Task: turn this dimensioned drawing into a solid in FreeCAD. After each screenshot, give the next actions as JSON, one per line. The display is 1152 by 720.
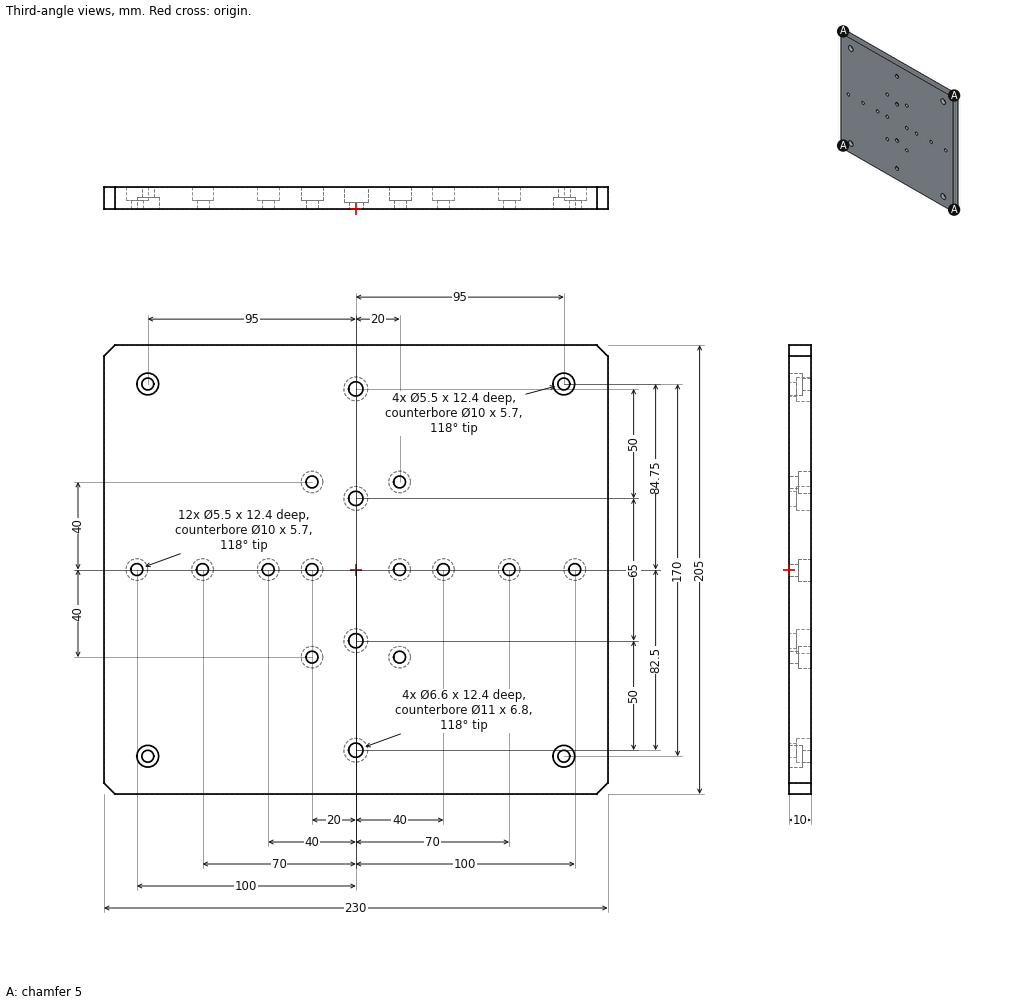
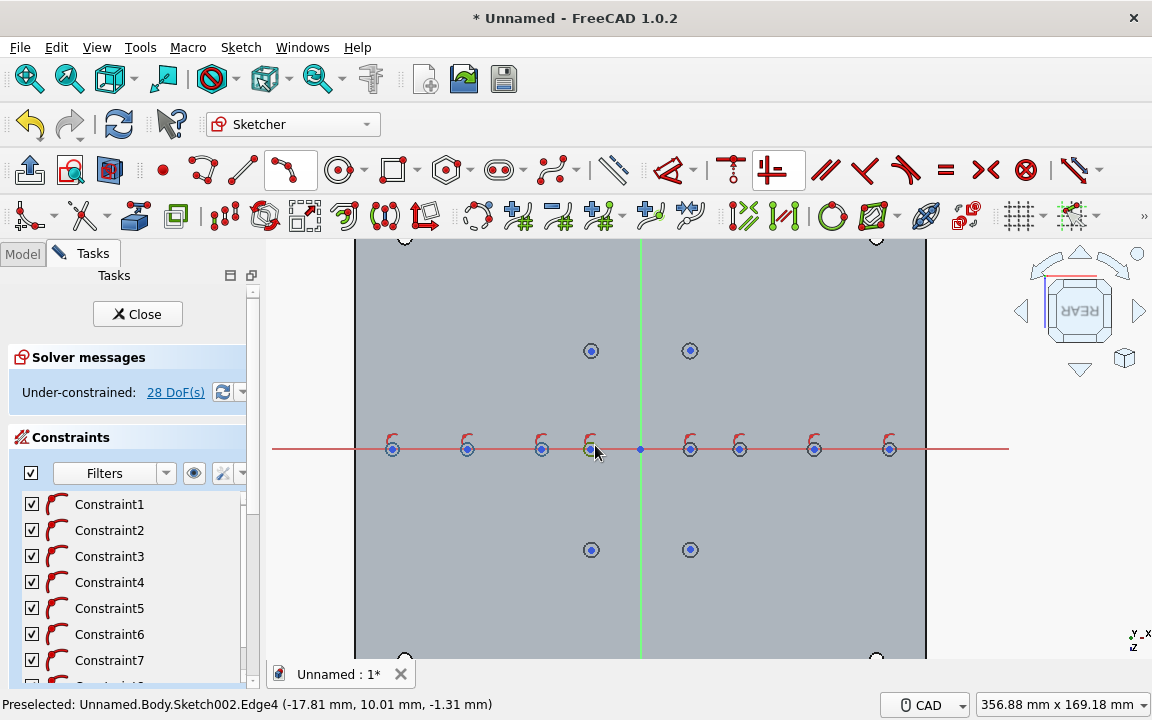
{"action": "scroll", "coordinate": [596, 346], "scroll_direction": "up", "scroll_amount": 4}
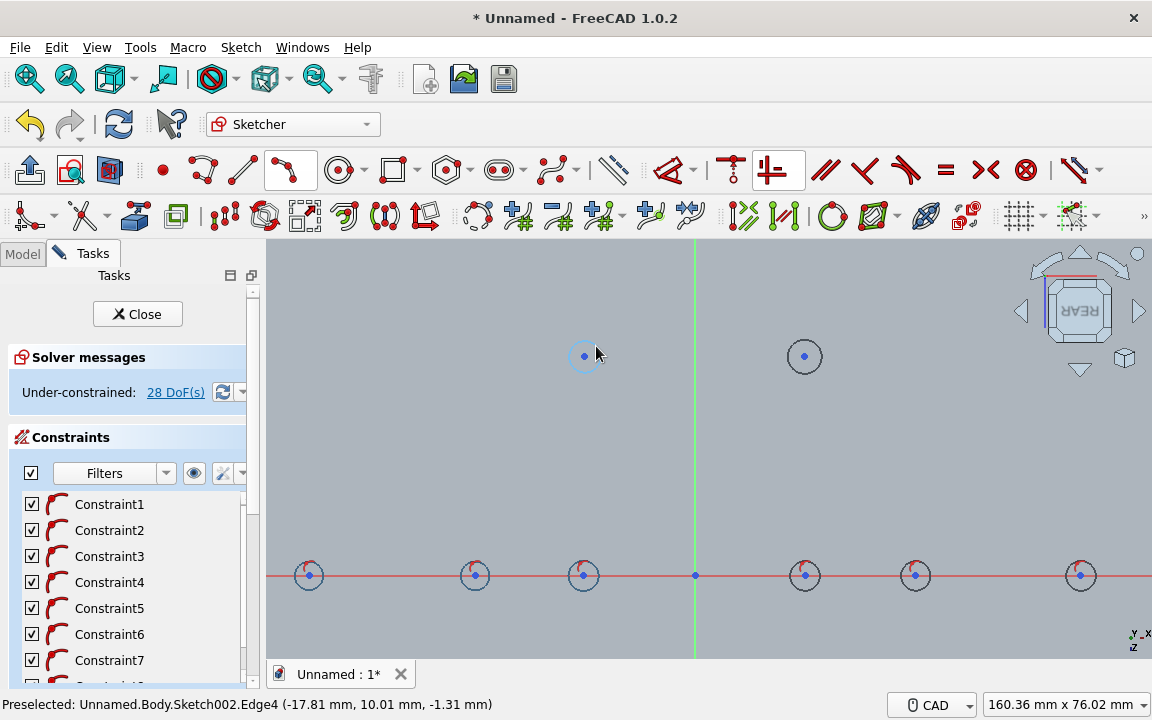
{"action": "left_click", "coordinate": [596, 346]}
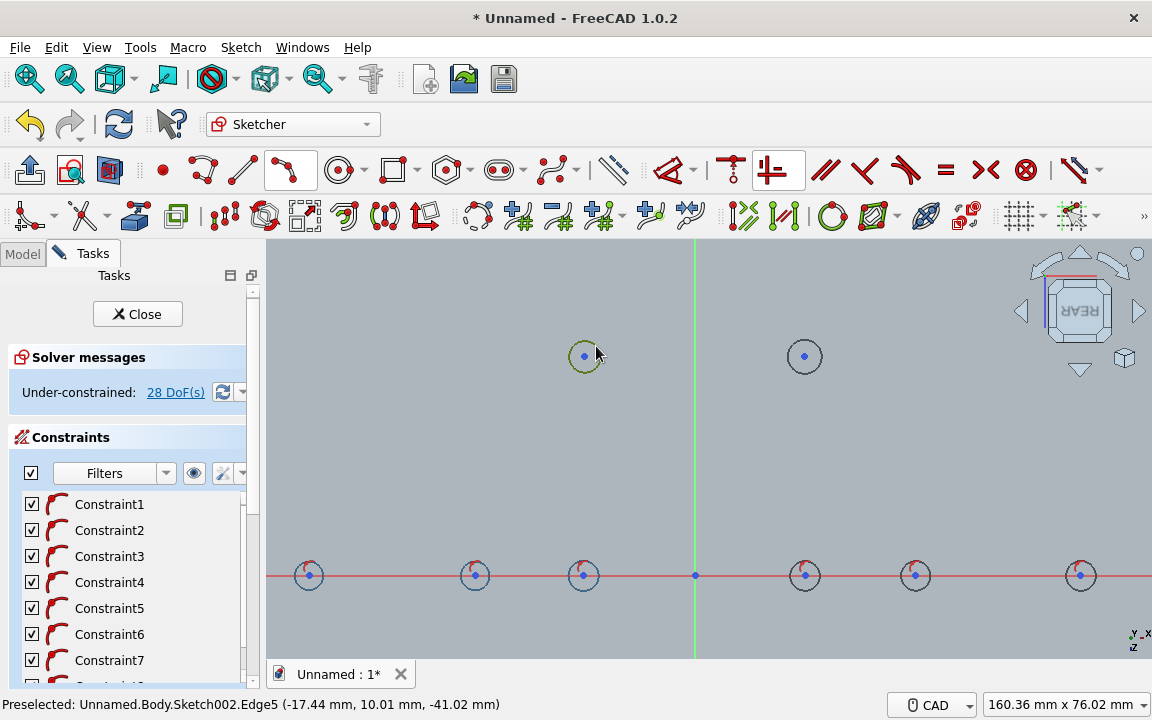
{"action": "scroll", "coordinate": [596, 345], "scroll_direction": "down", "scroll_amount": 4}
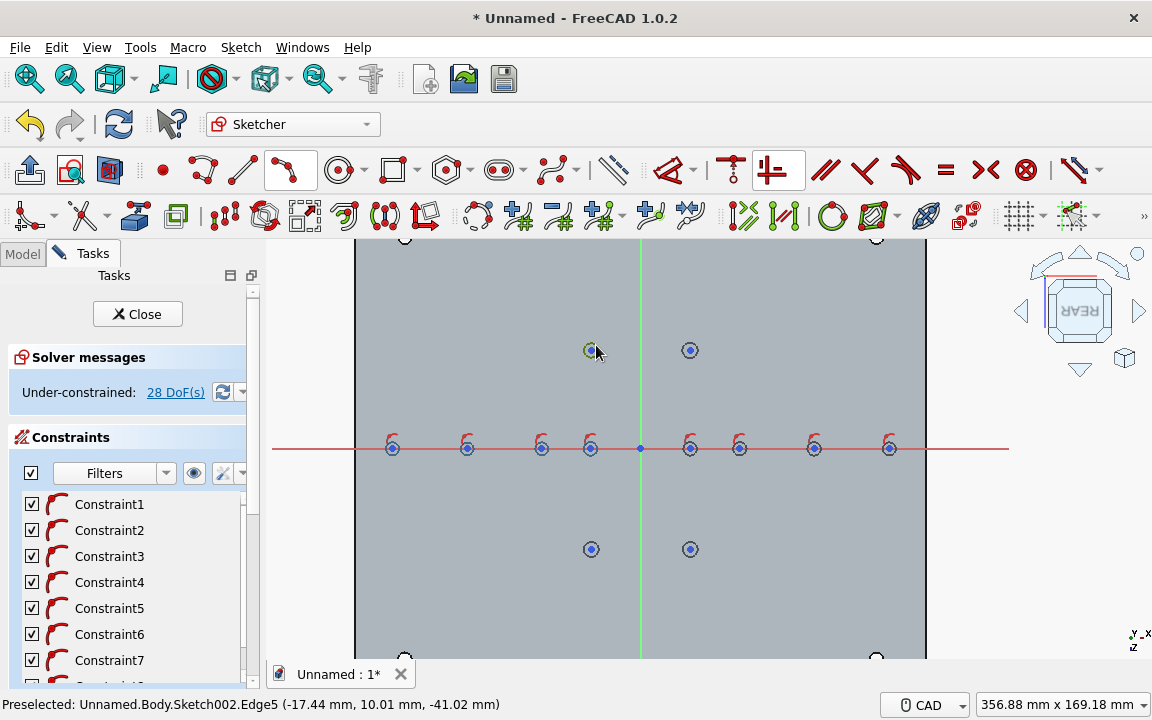
{"action": "scroll", "coordinate": [596, 544], "scroll_direction": "up", "scroll_amount": 4}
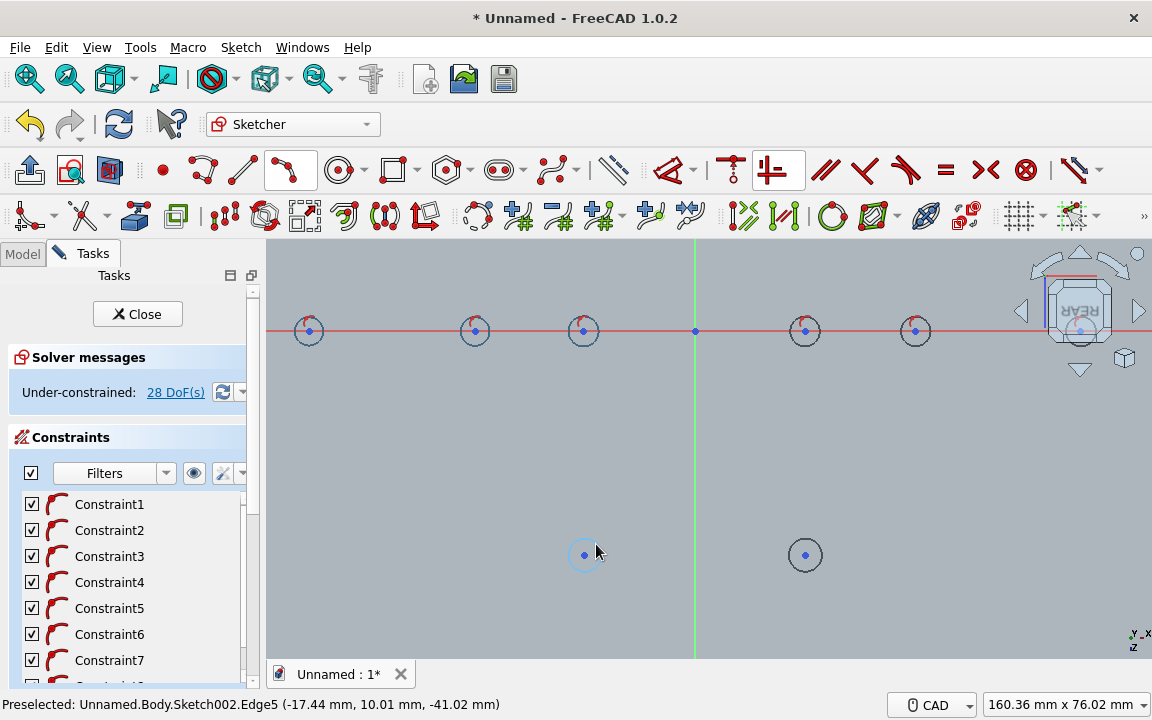
{"action": "left_click", "coordinate": [597, 544]}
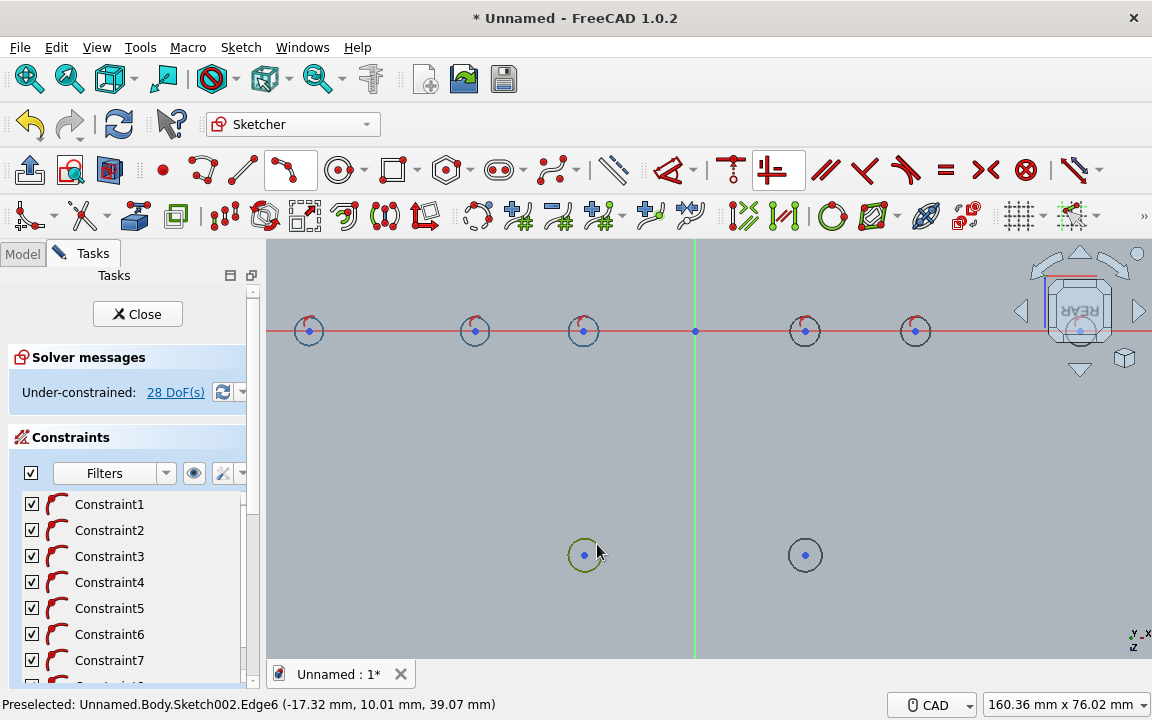
{"action": "left_click", "coordinate": [817, 543]}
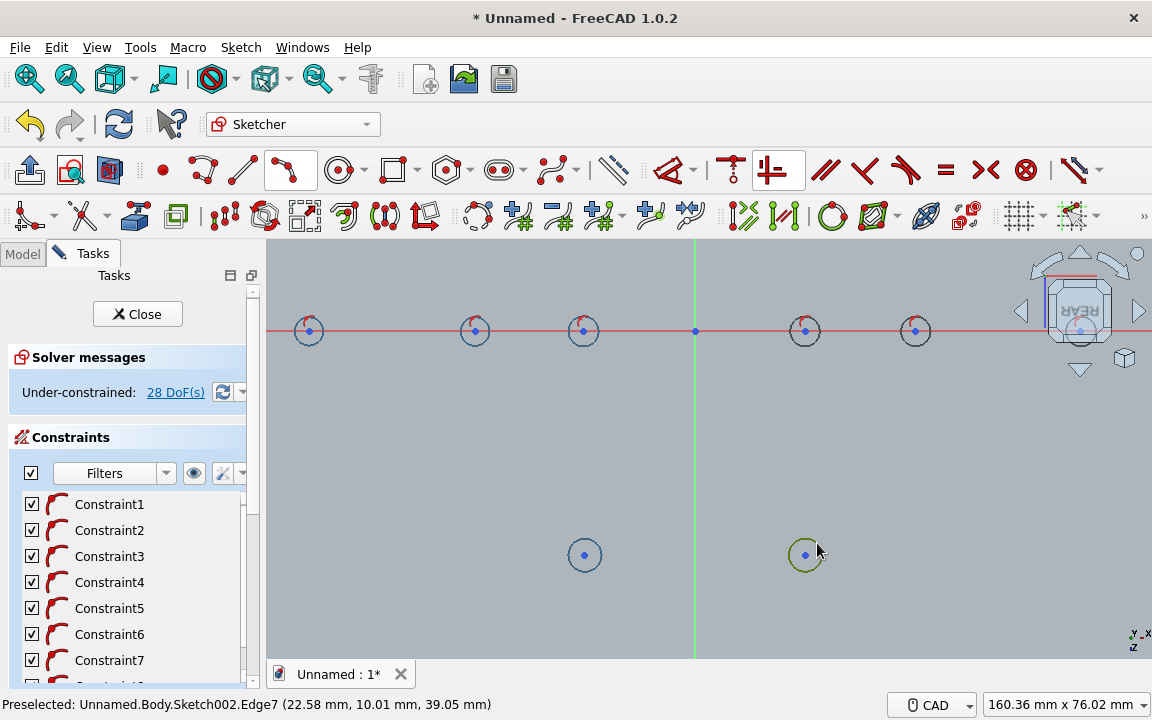
{"action": "scroll", "coordinate": [926, 321], "scroll_direction": "up", "scroll_amount": 2}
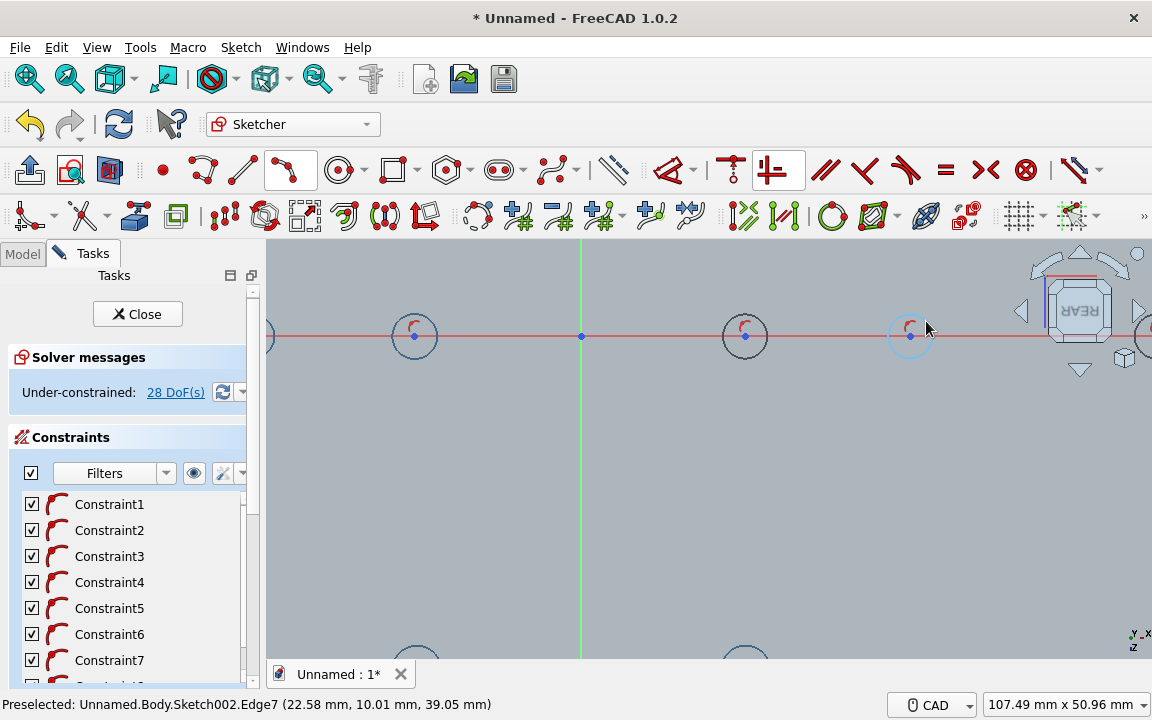
{"action": "left_click", "coordinate": [926, 321]}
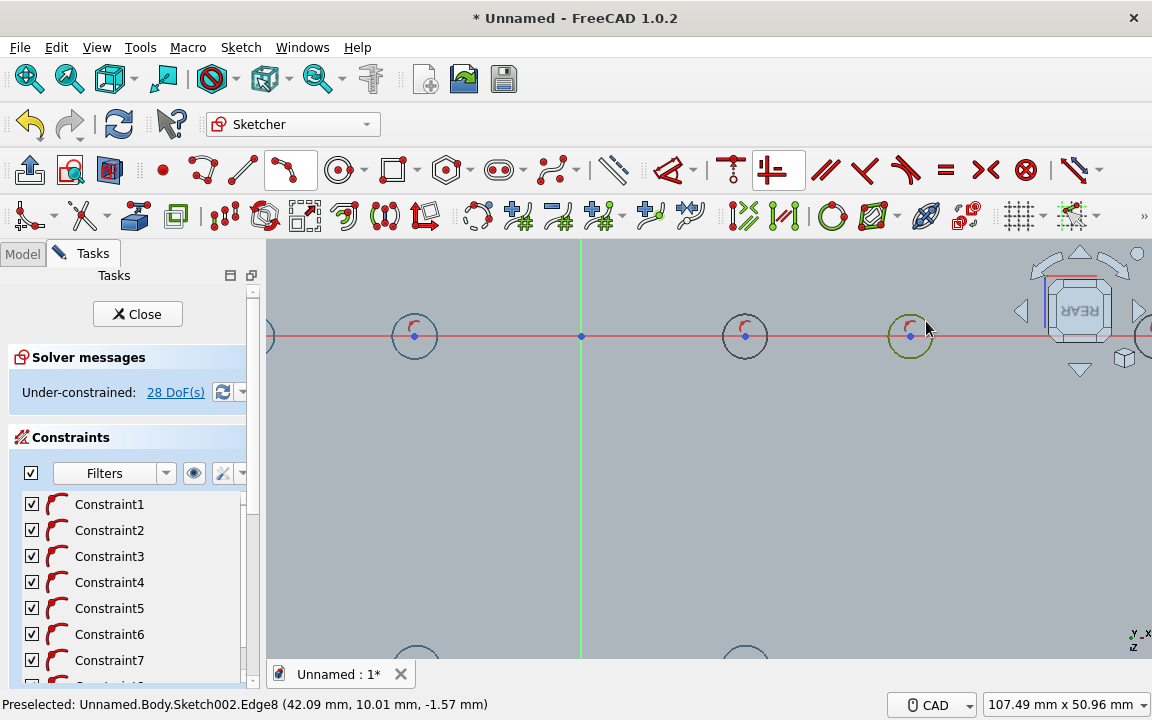
{"action": "left_click", "coordinate": [761, 321]}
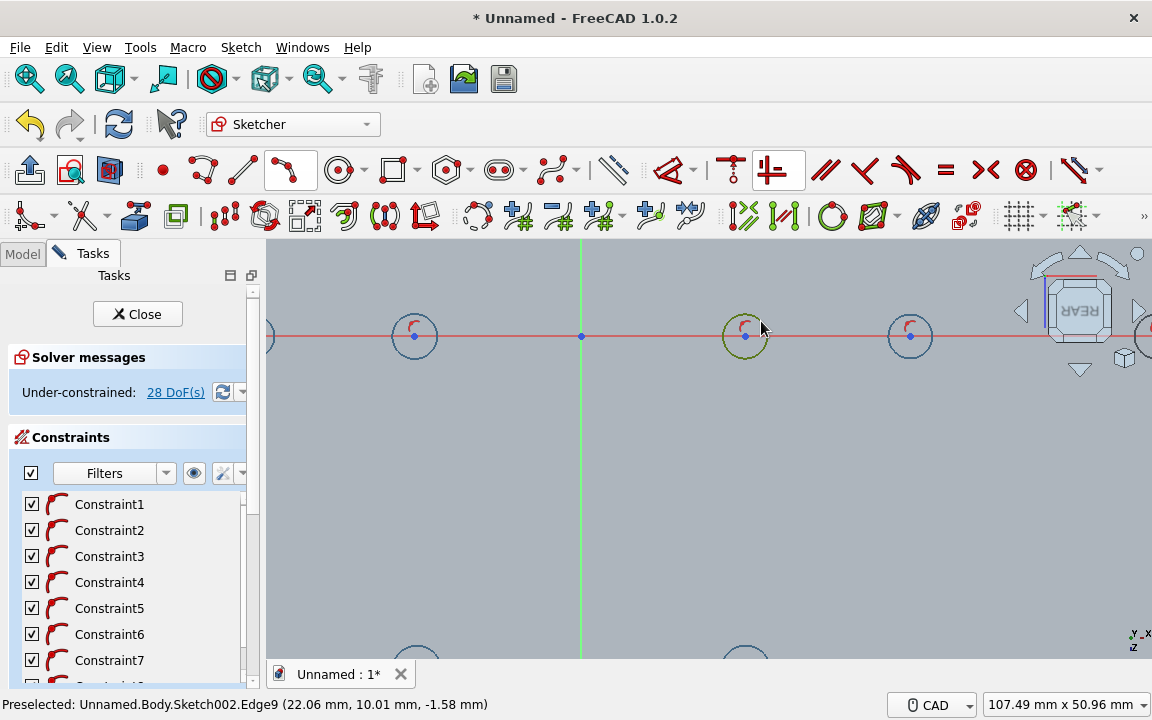
{"action": "scroll", "coordinate": [666, 497], "scroll_direction": "down", "scroll_amount": 6}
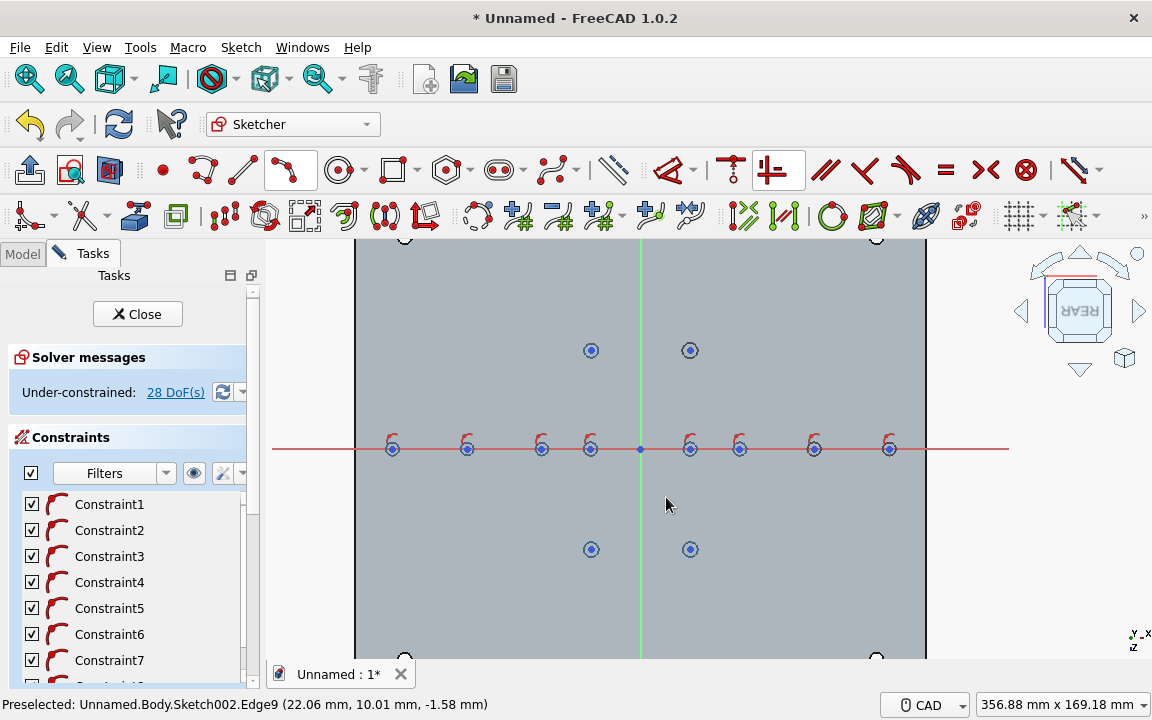
{"action": "scroll", "coordinate": [819, 444], "scroll_direction": "up", "scroll_amount": 6}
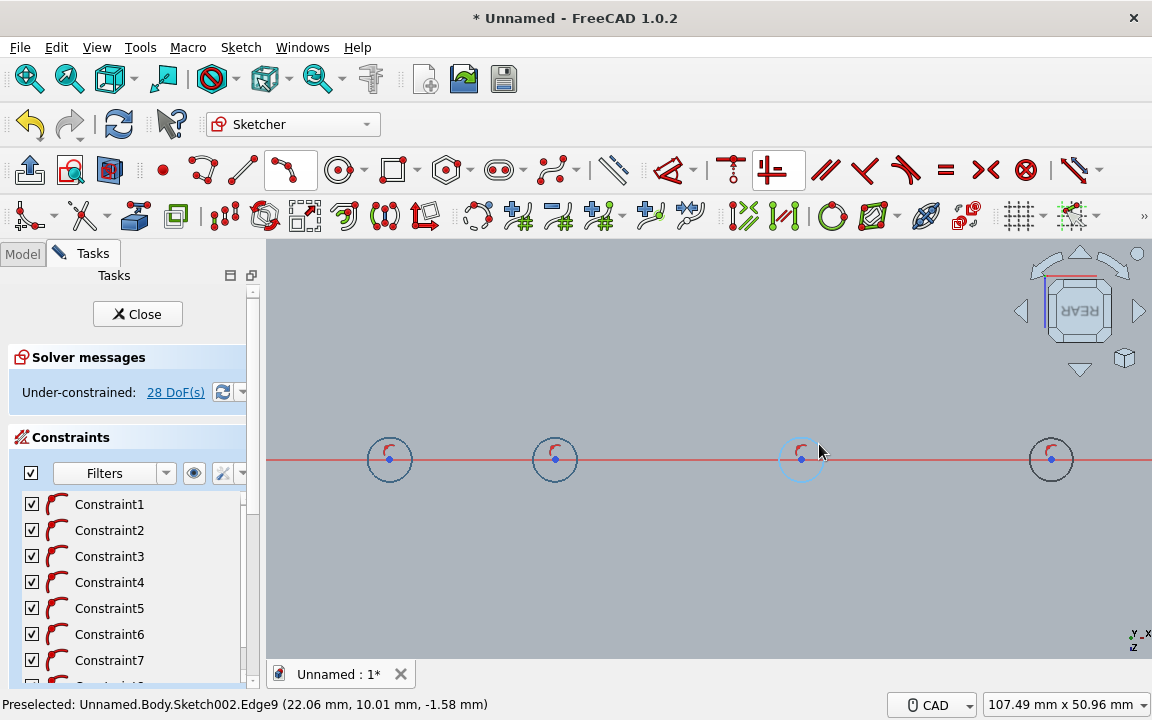
{"action": "left_click", "coordinate": [817, 444]}